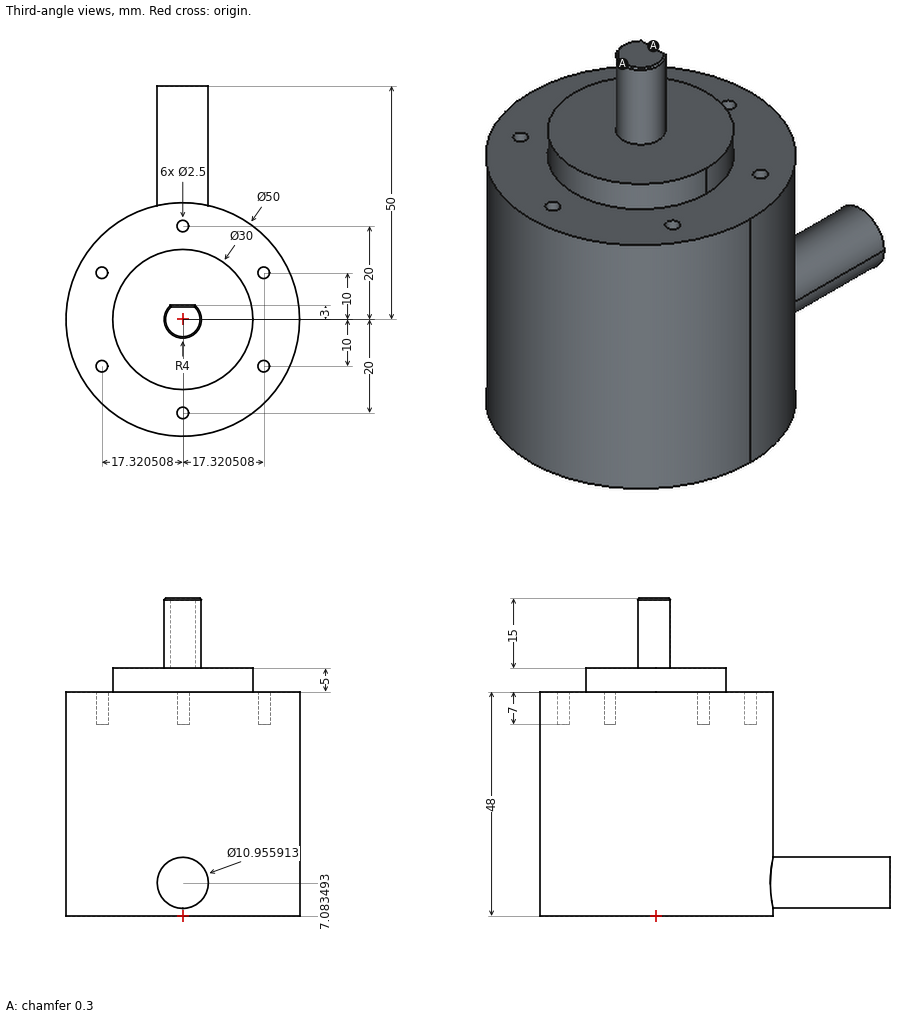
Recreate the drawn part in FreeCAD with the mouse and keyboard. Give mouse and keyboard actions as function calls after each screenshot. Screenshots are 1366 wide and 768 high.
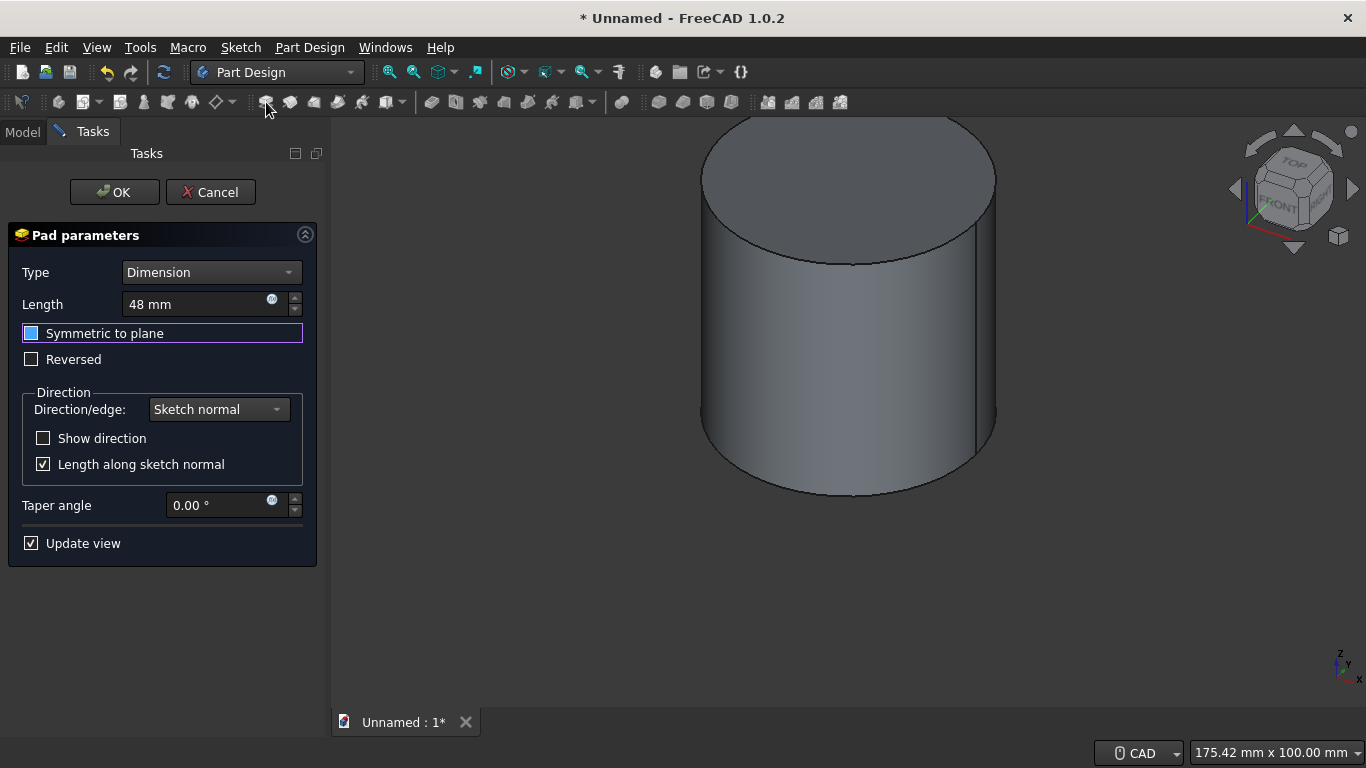
click(115, 192)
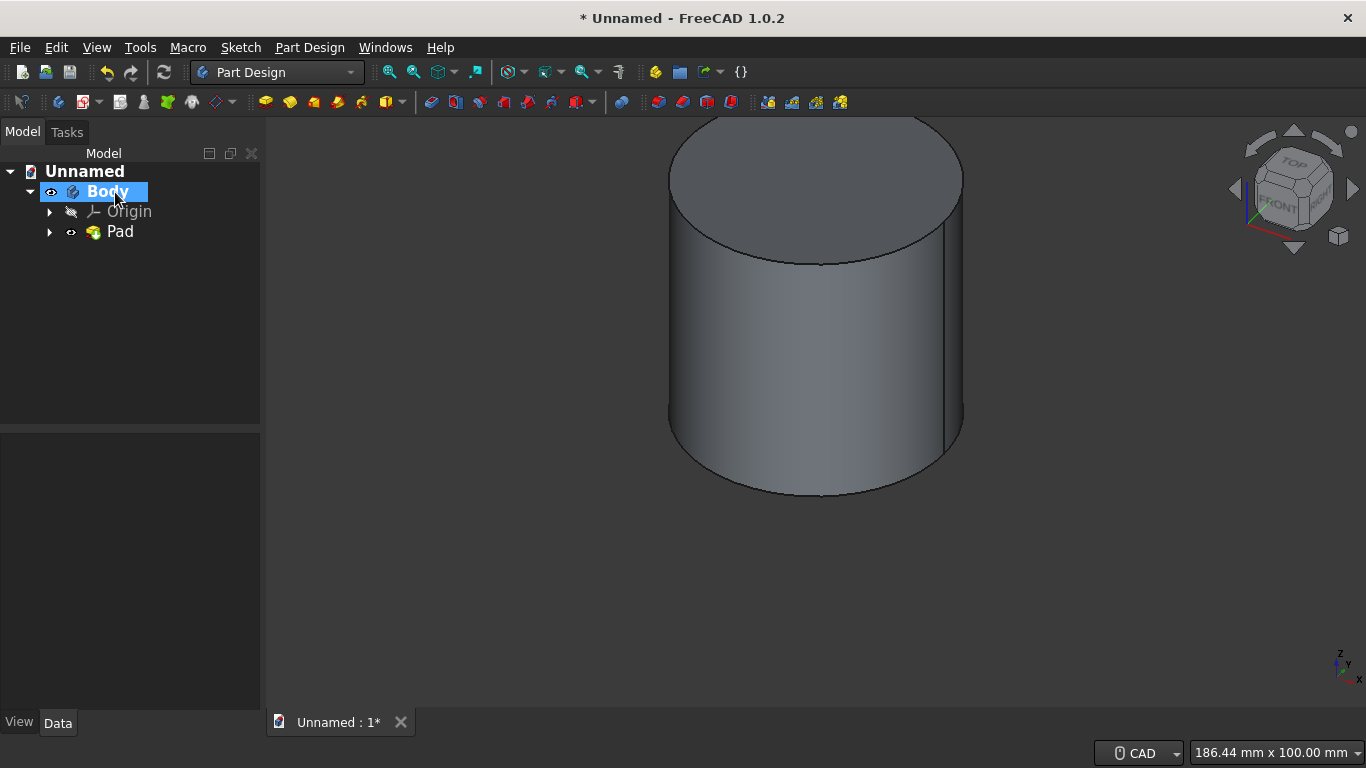
click(390, 72)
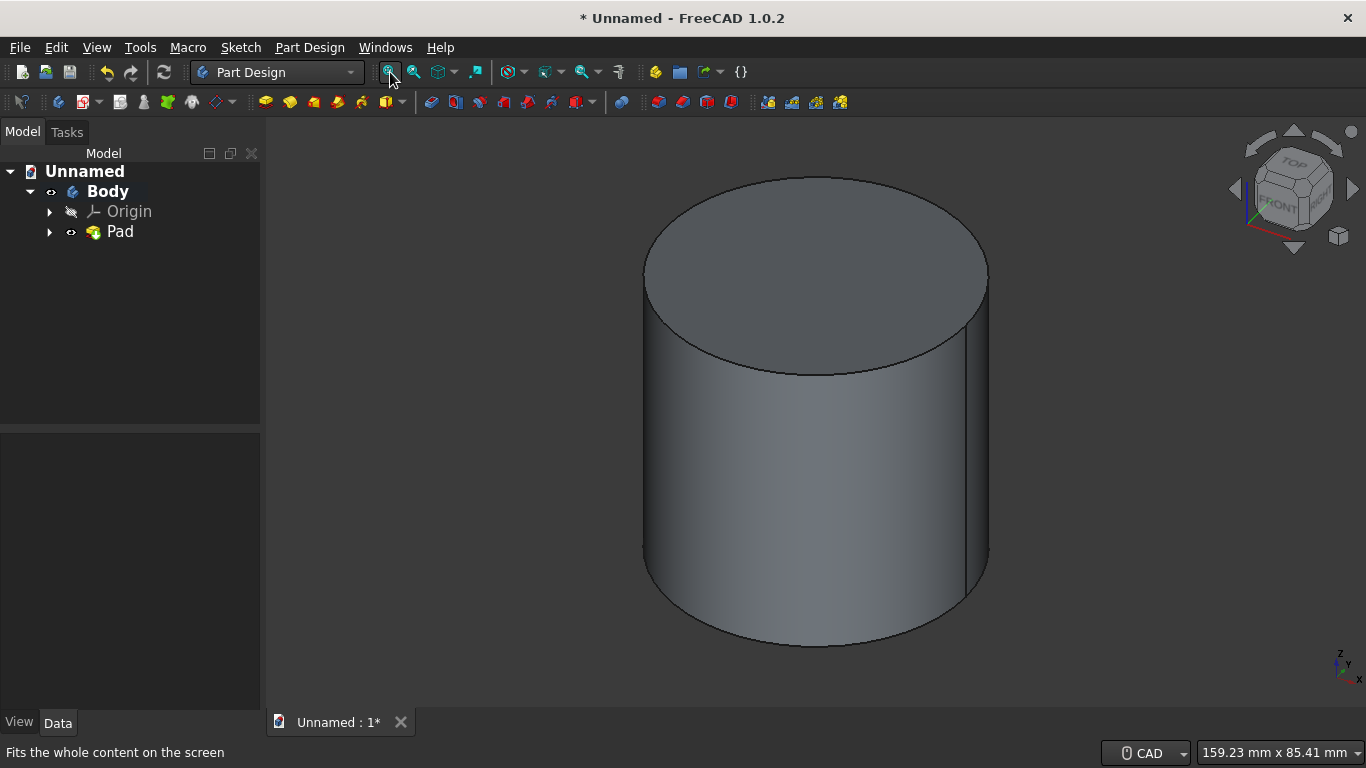
click(816, 275)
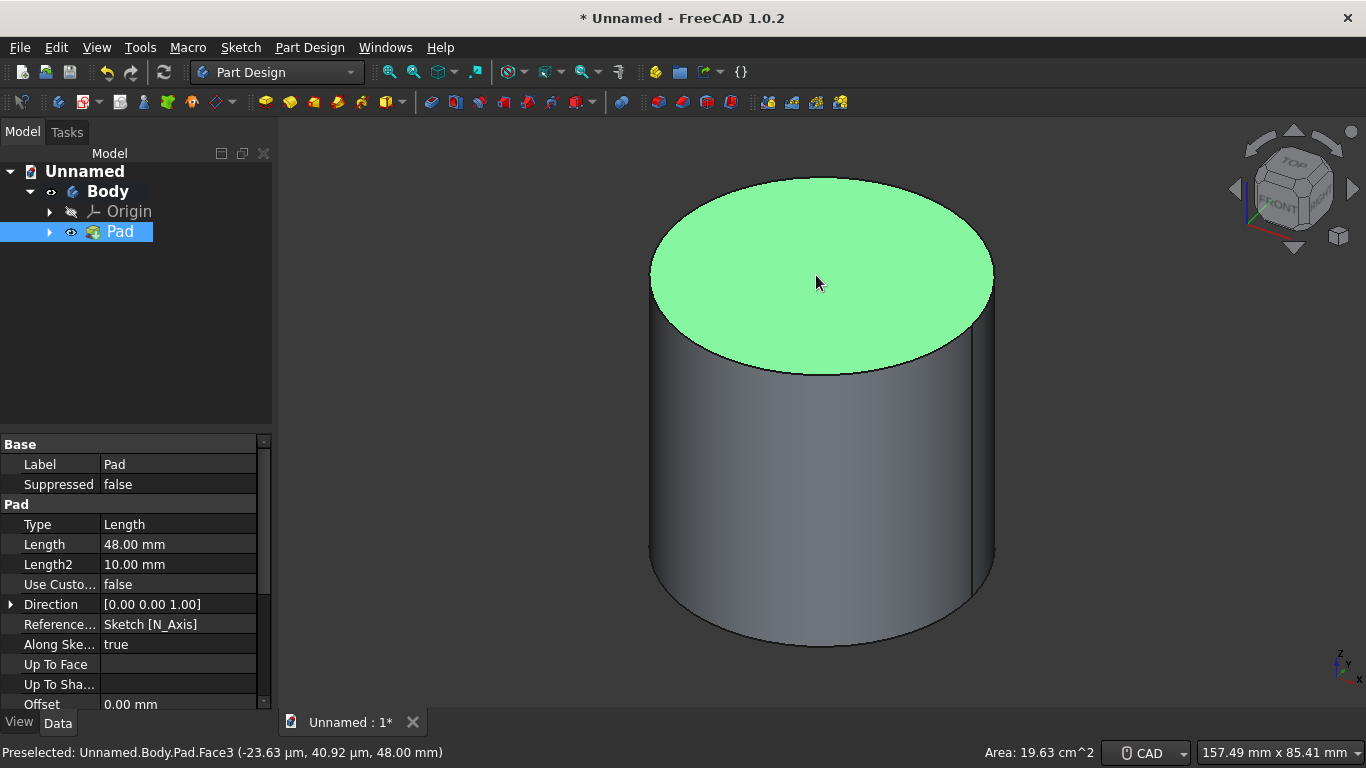
click(84, 102)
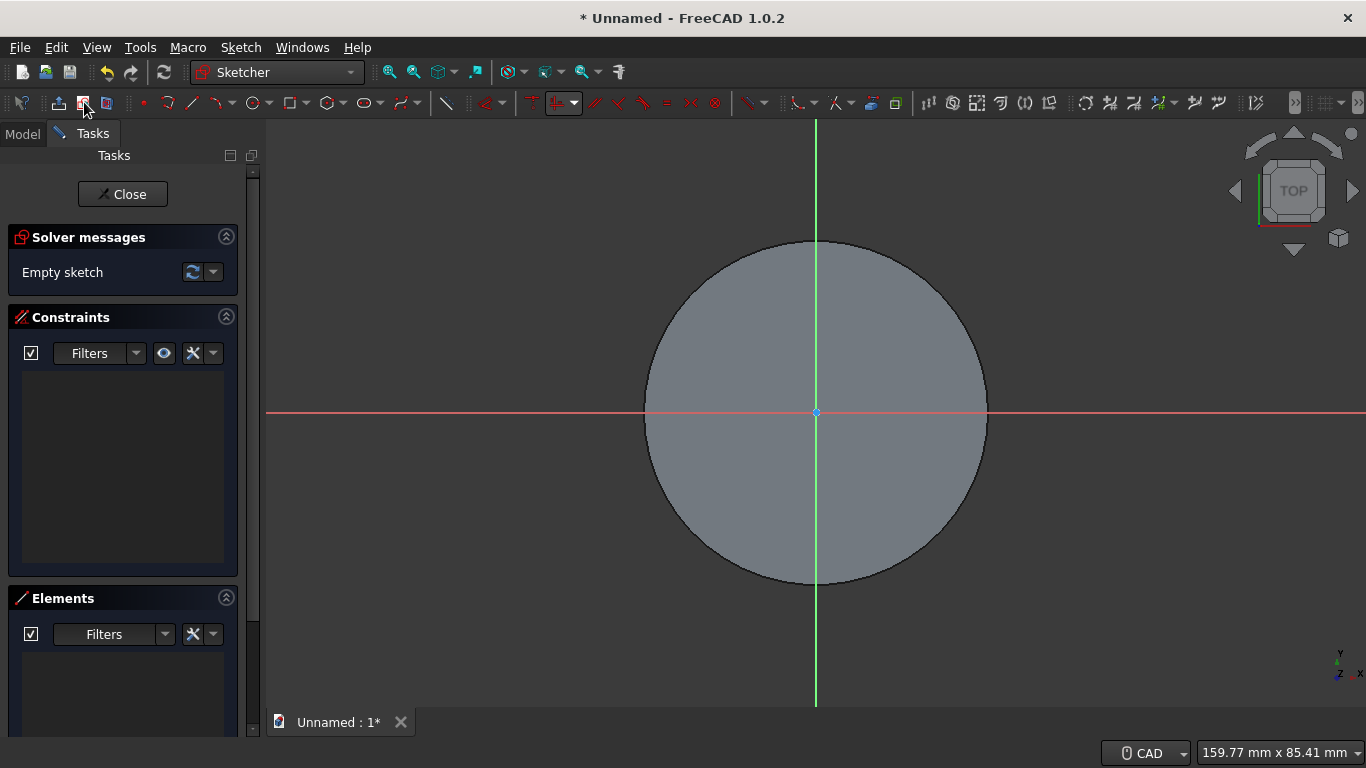
scroll(899, 413, up, 3)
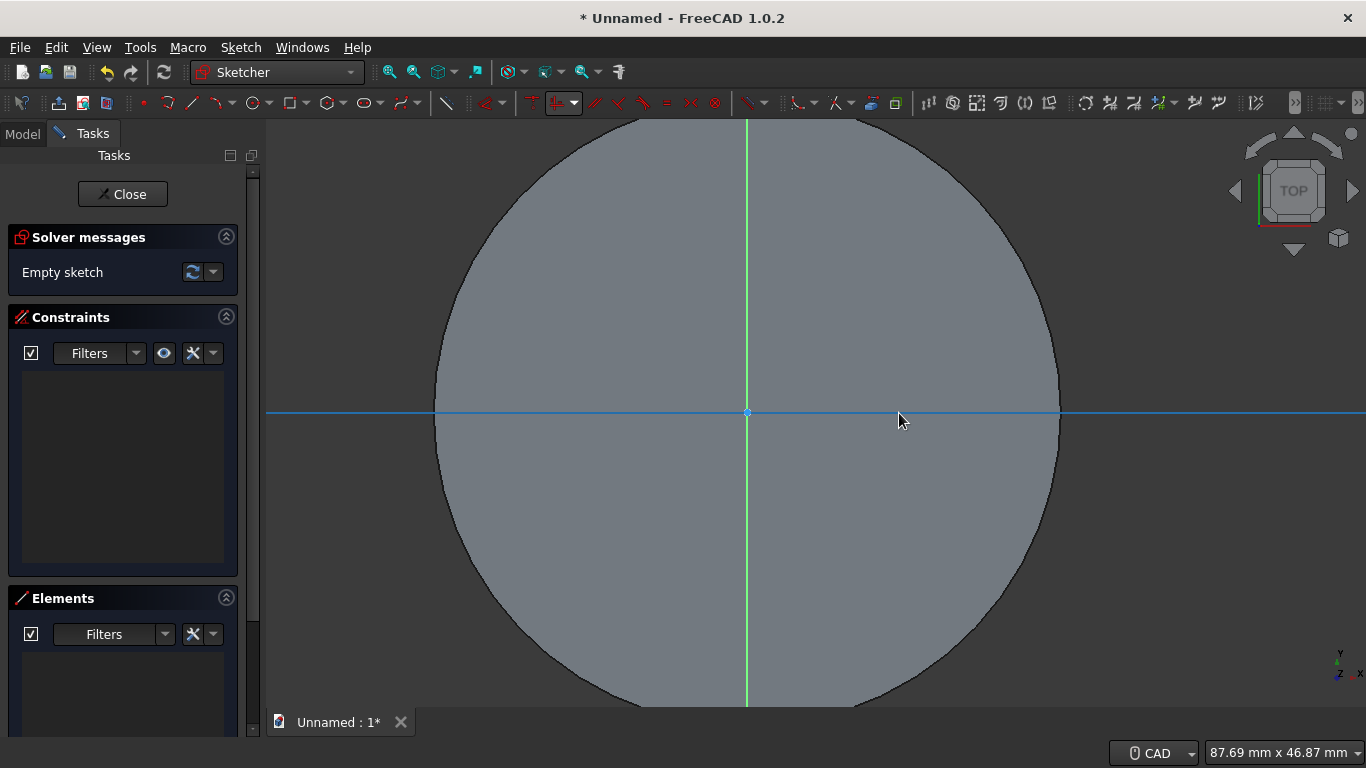
click(254, 104)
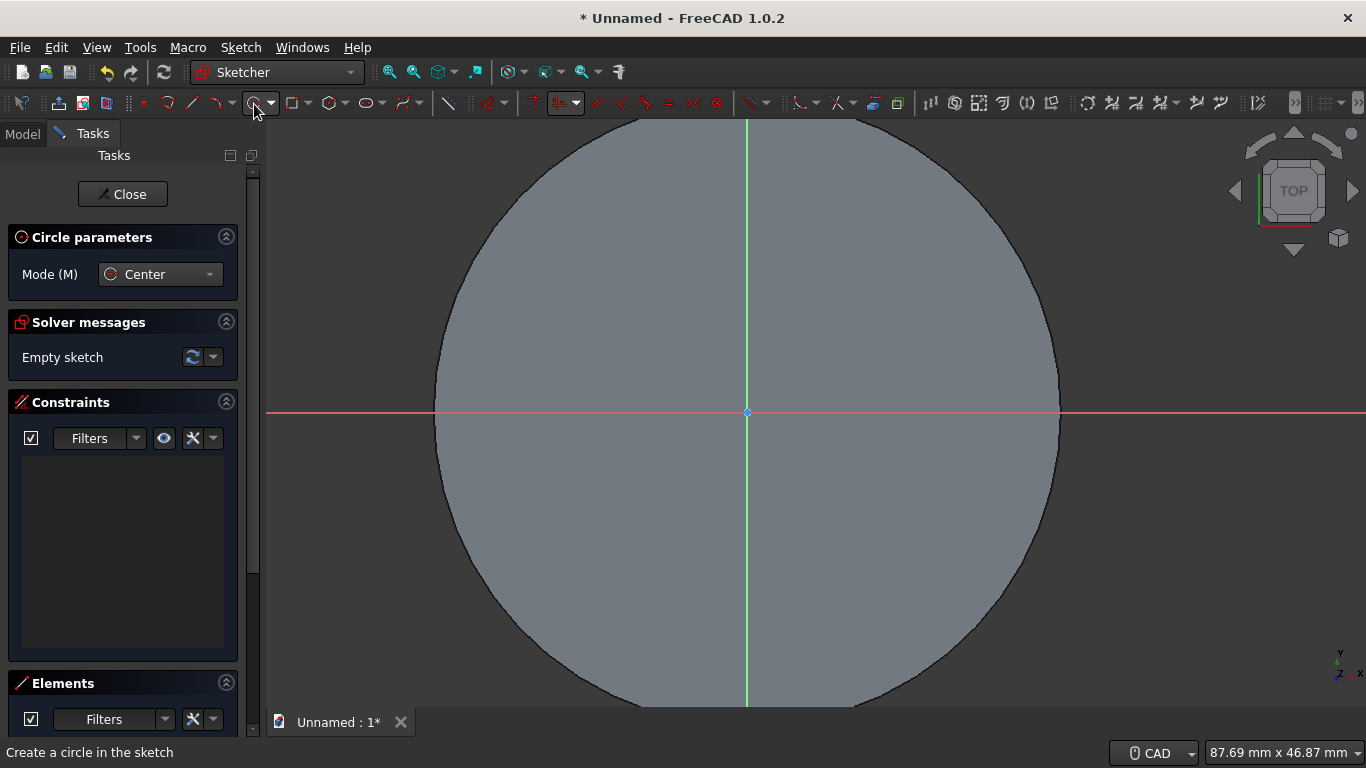
click(747, 413)
move(880, 280)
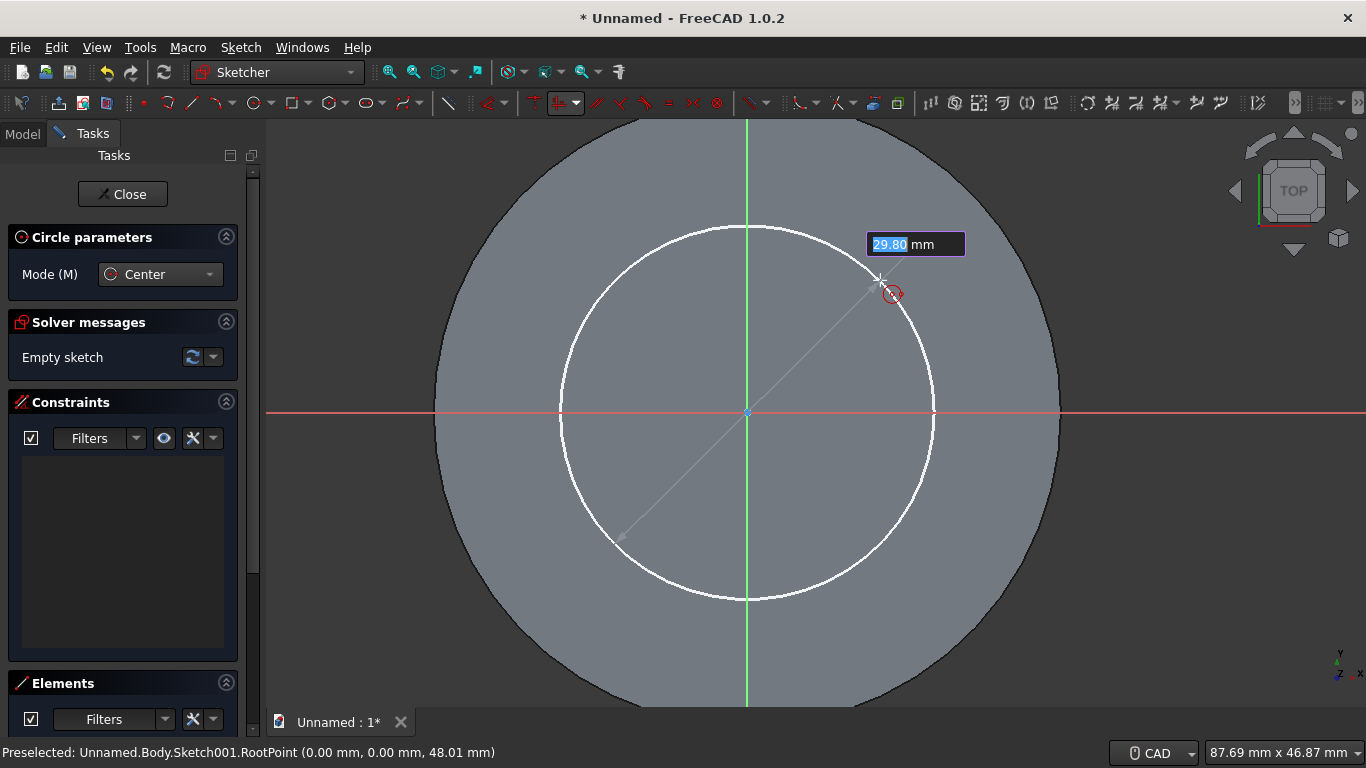
text(30)
key(Return)
key(Escape)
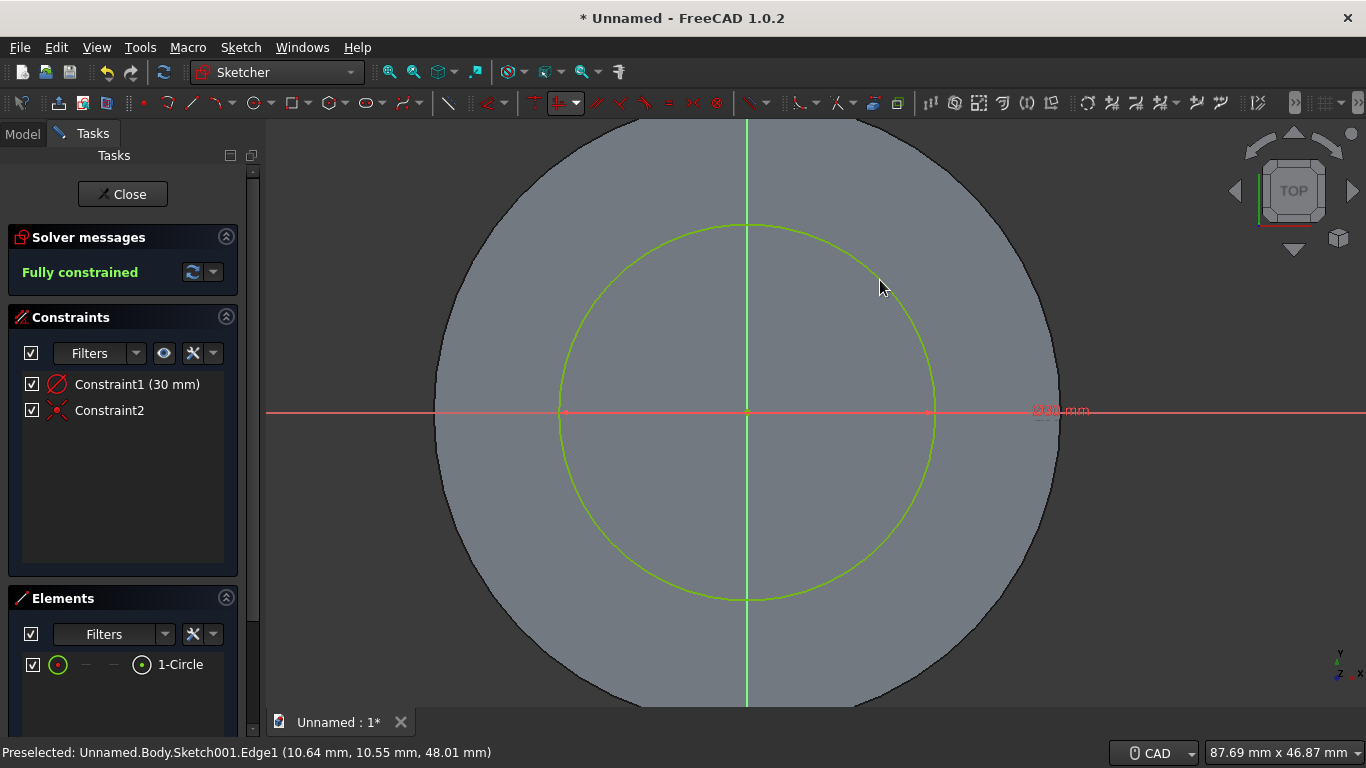
click(123, 194)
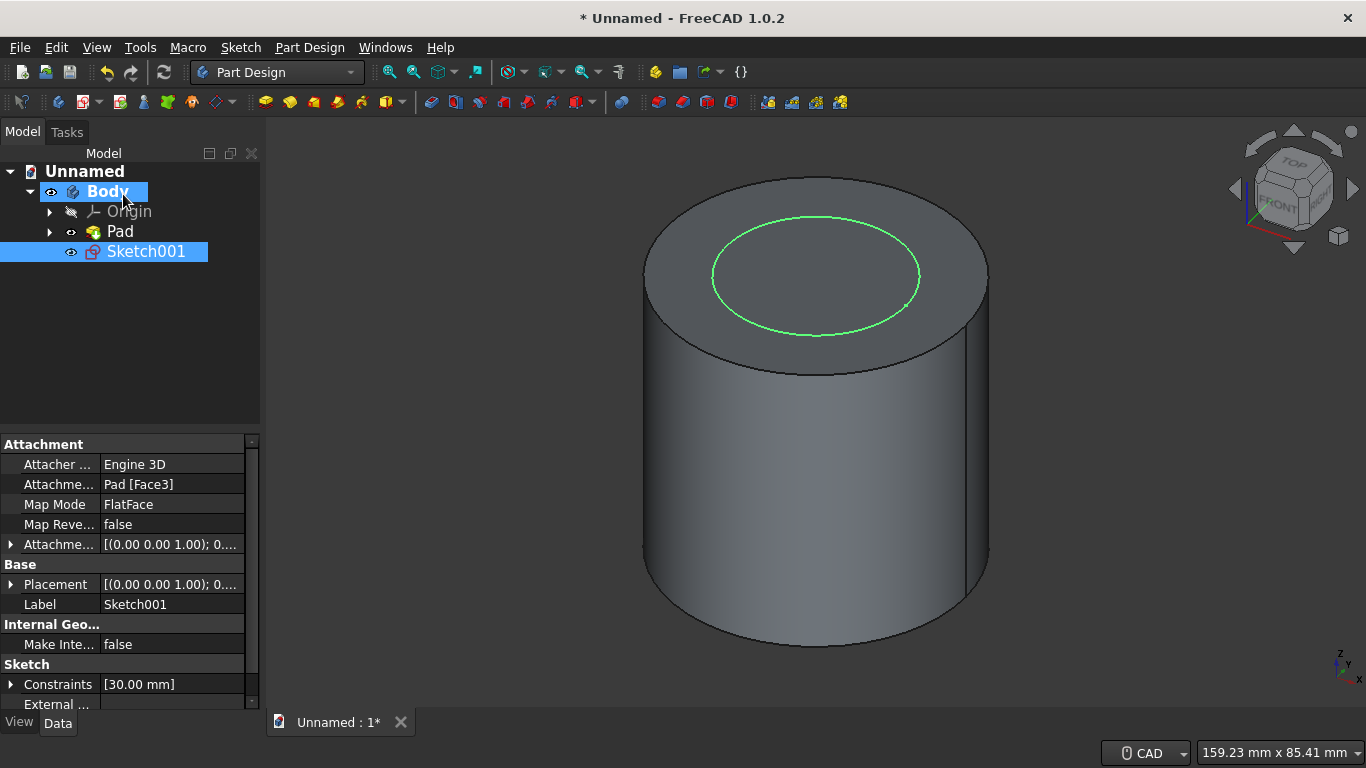
click(266, 102)